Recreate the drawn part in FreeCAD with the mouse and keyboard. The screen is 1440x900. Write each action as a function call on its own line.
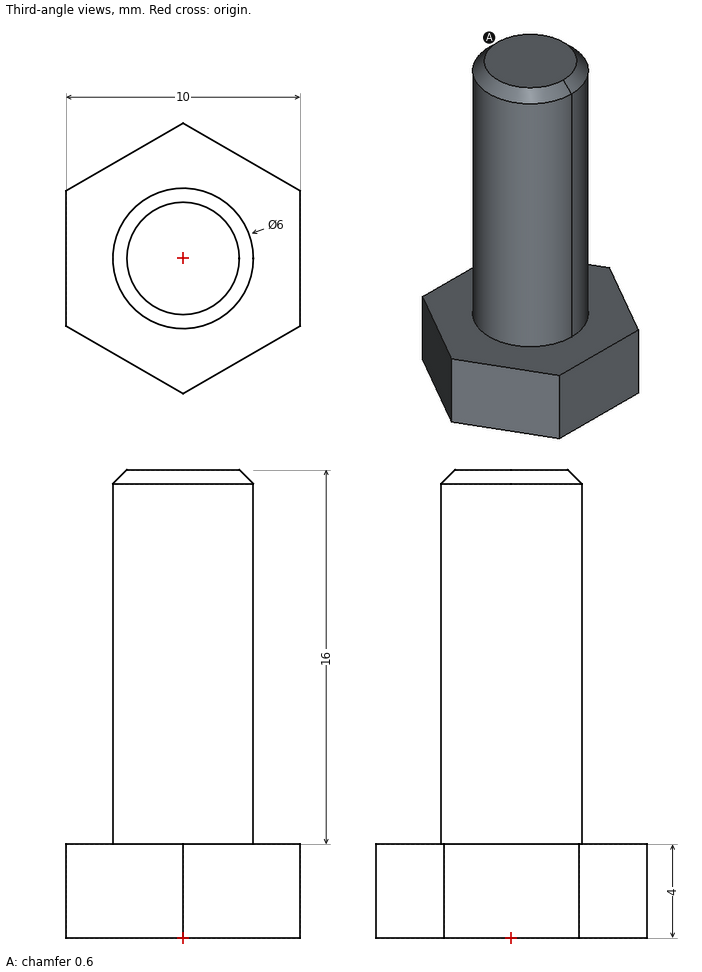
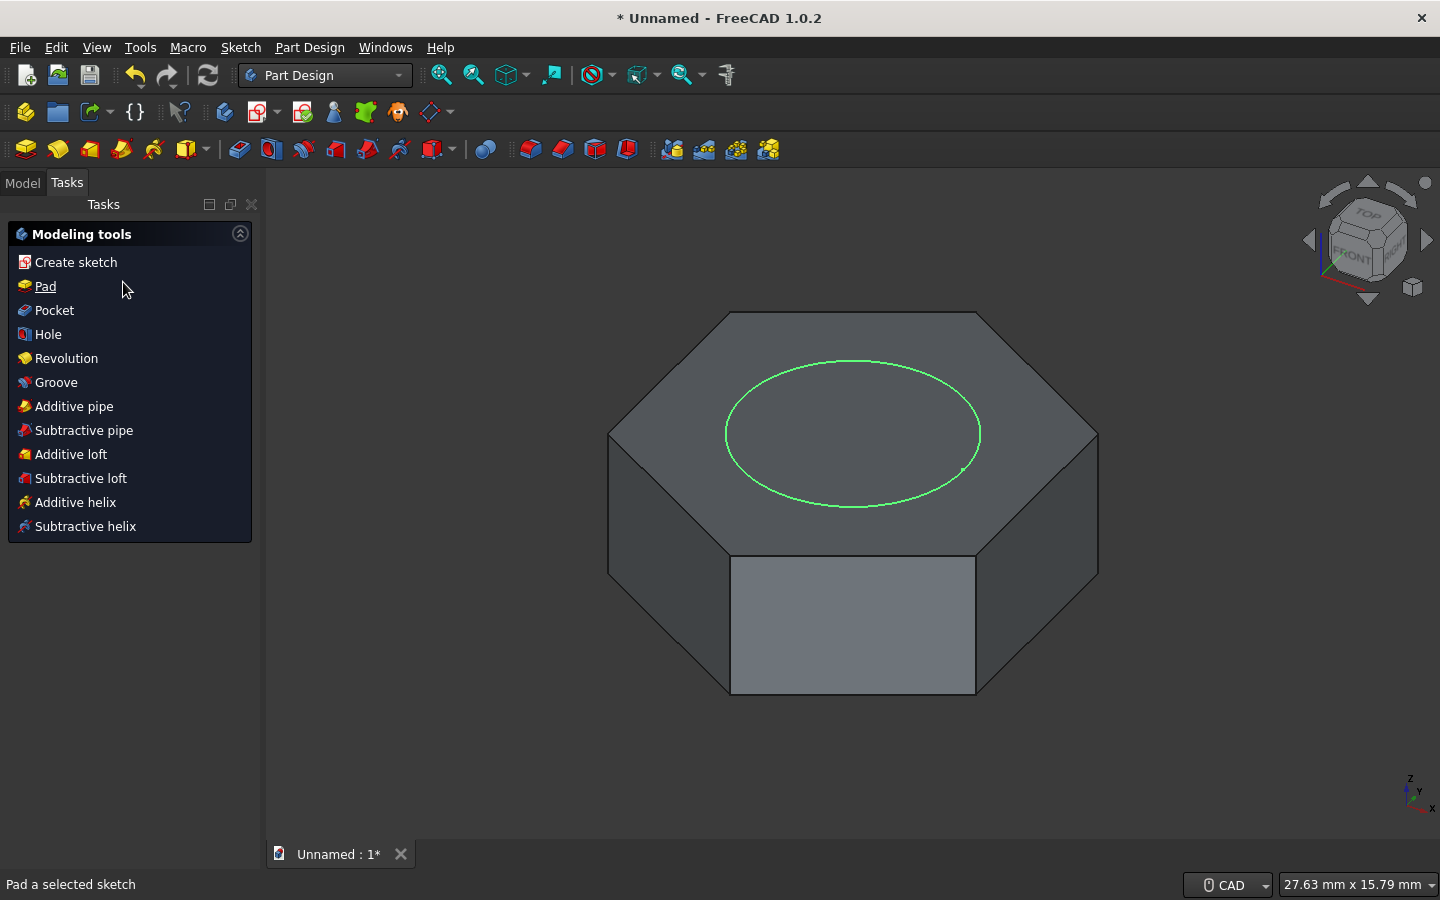
click(26, 150)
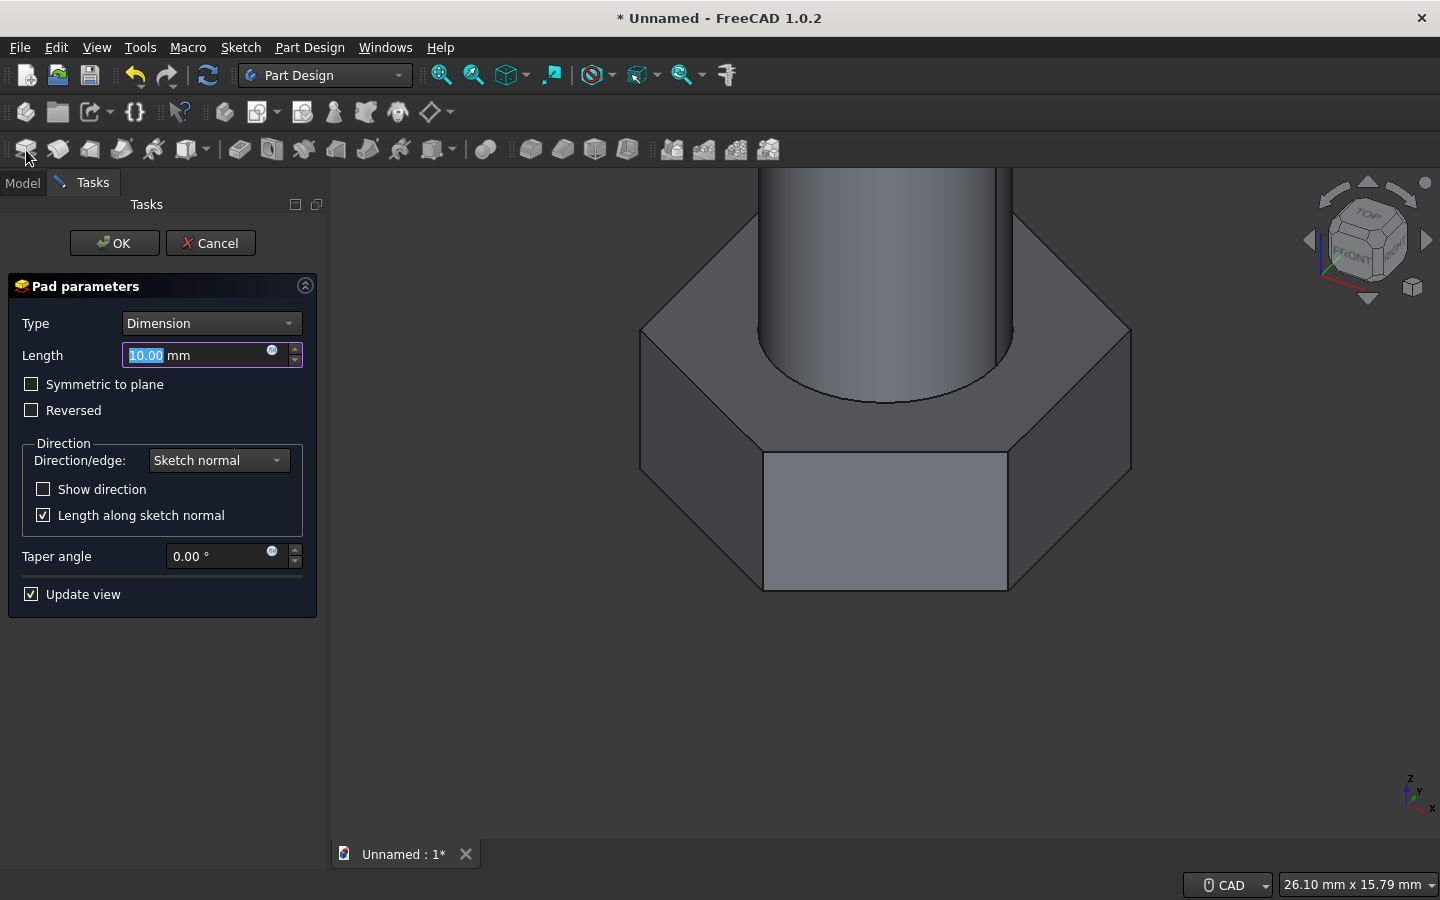
text(16)
key(Tab)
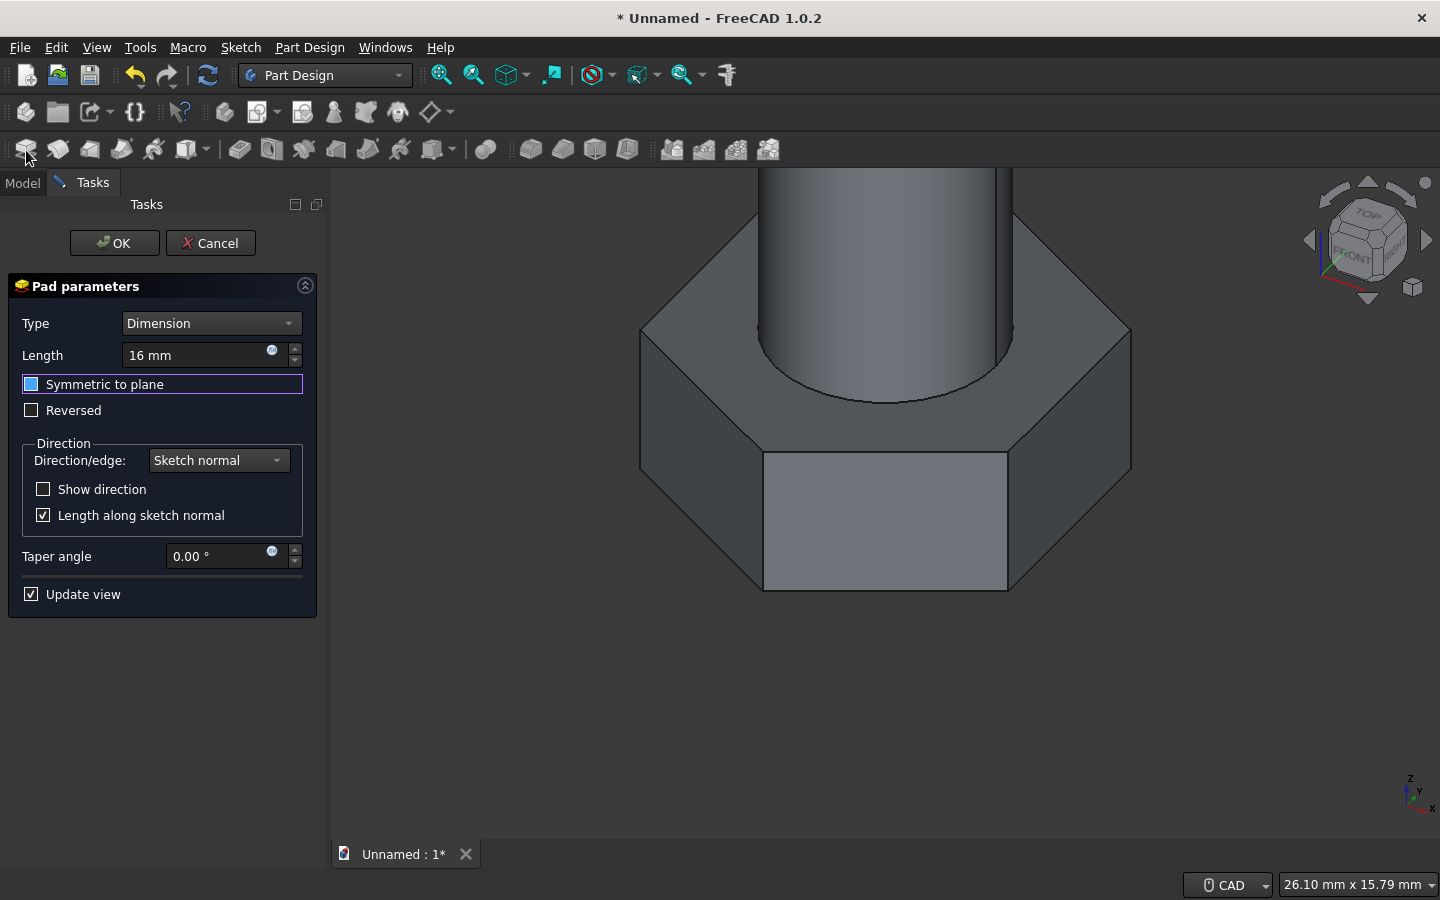
click(115, 243)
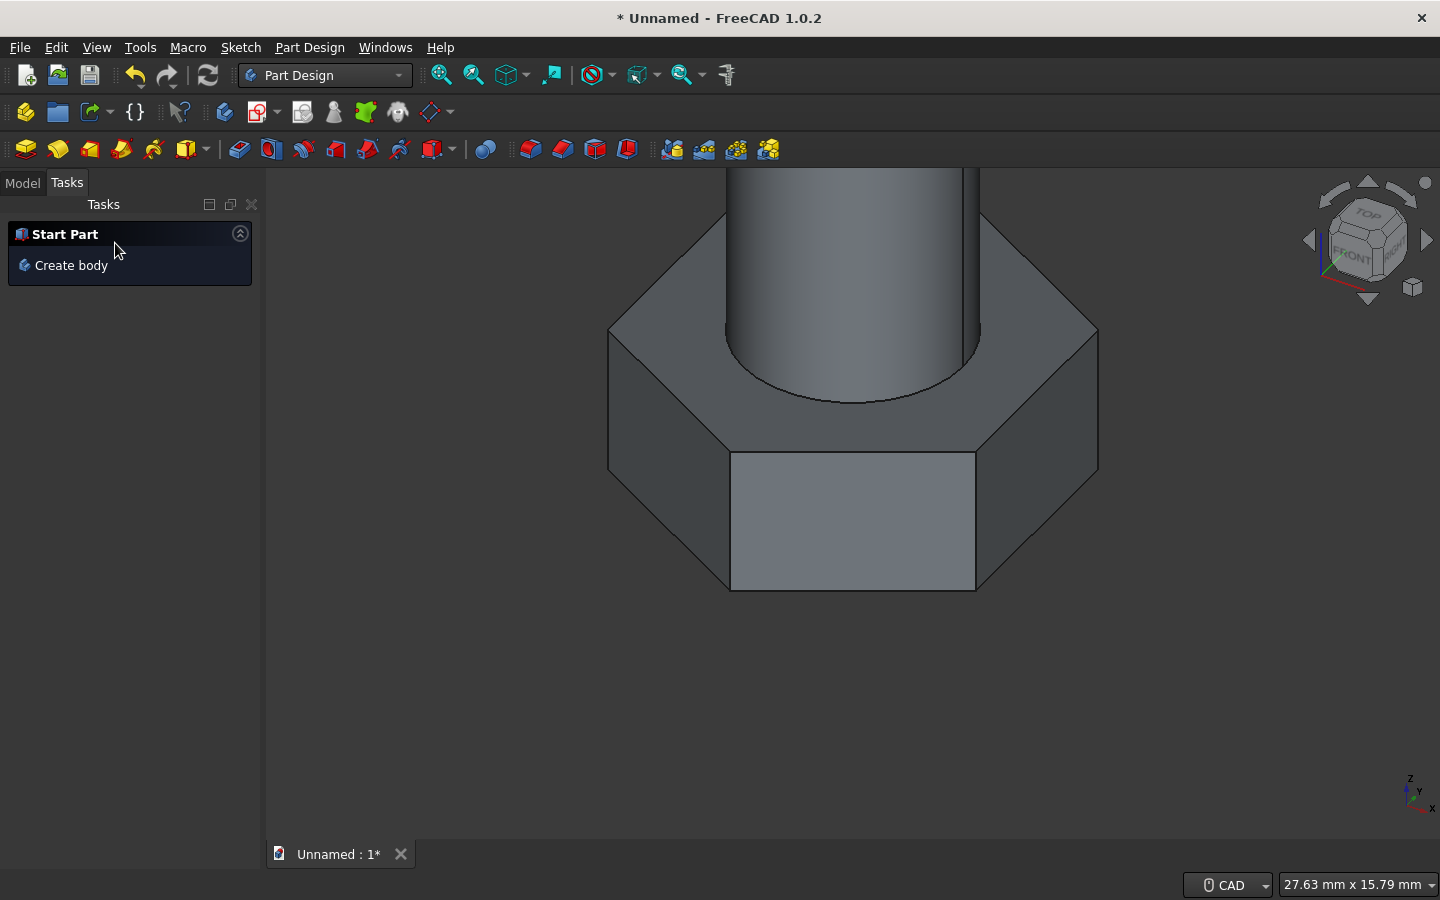
click(442, 76)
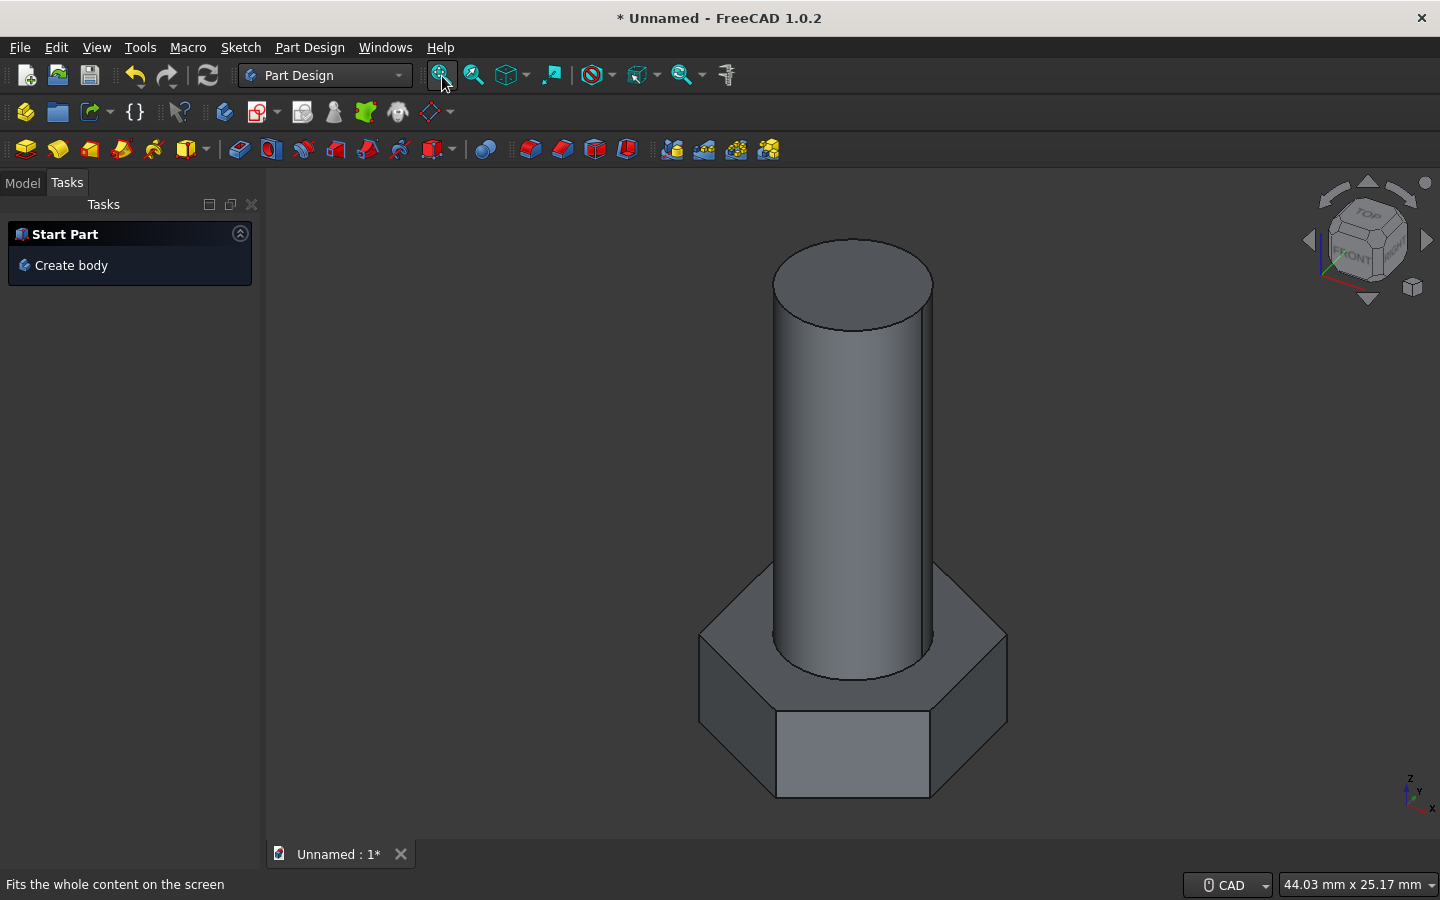
click(773, 289)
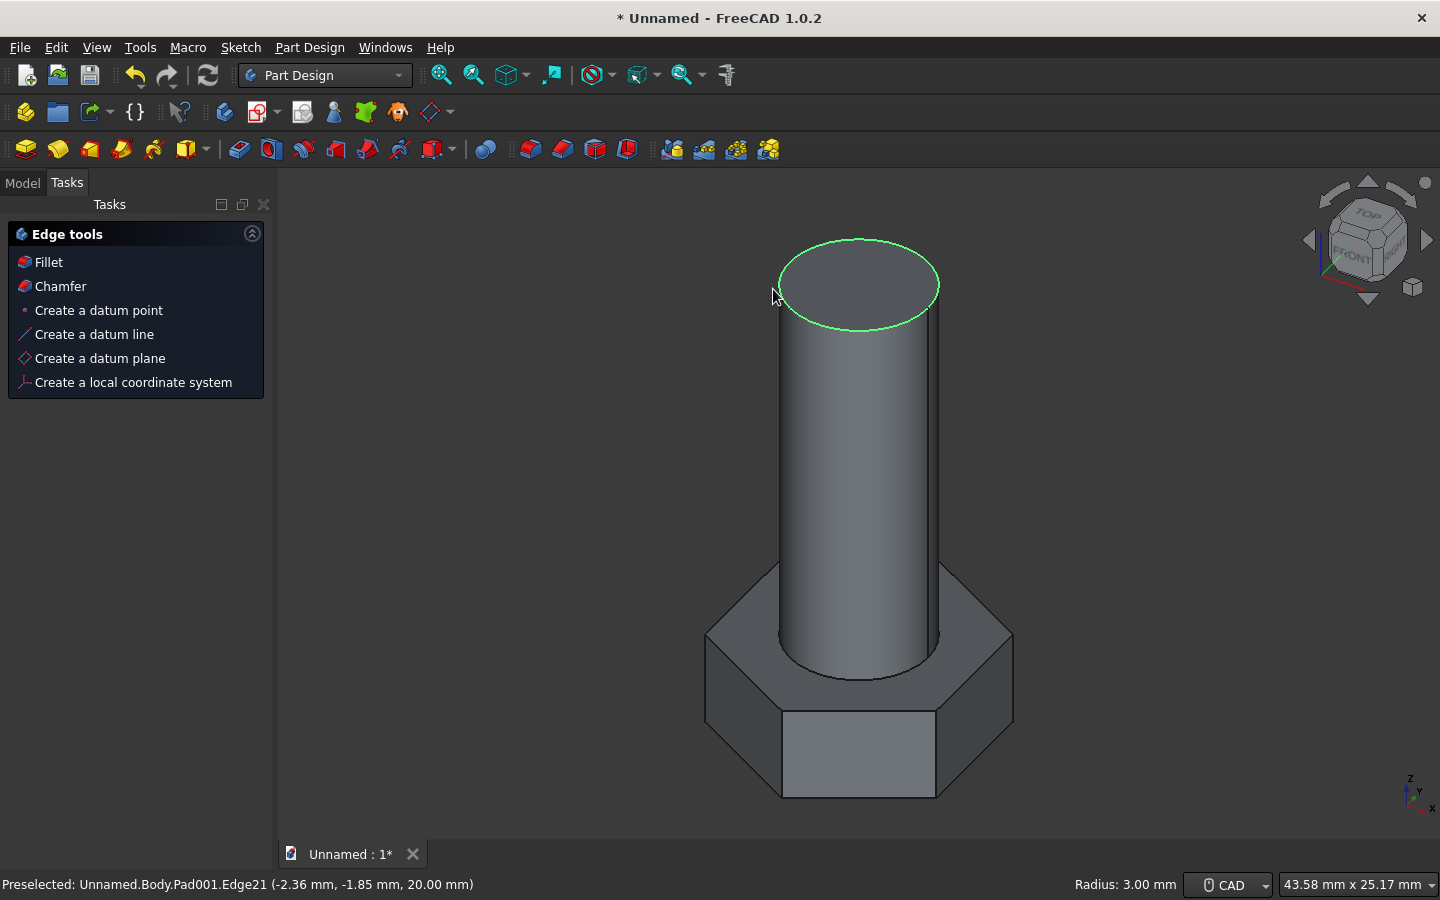
click(564, 150)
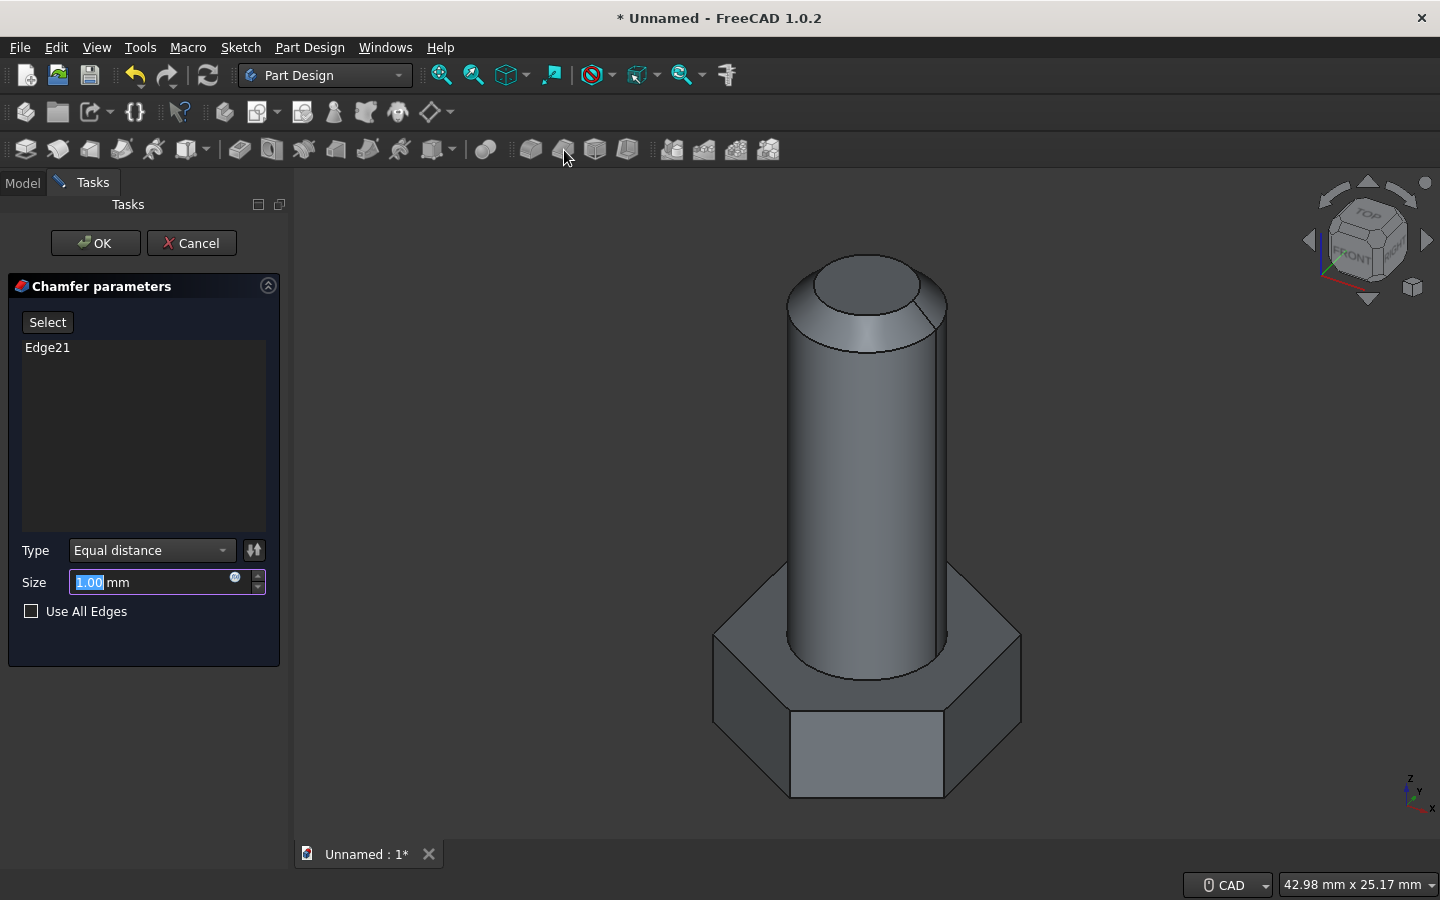
text(0.6)
key(Tab)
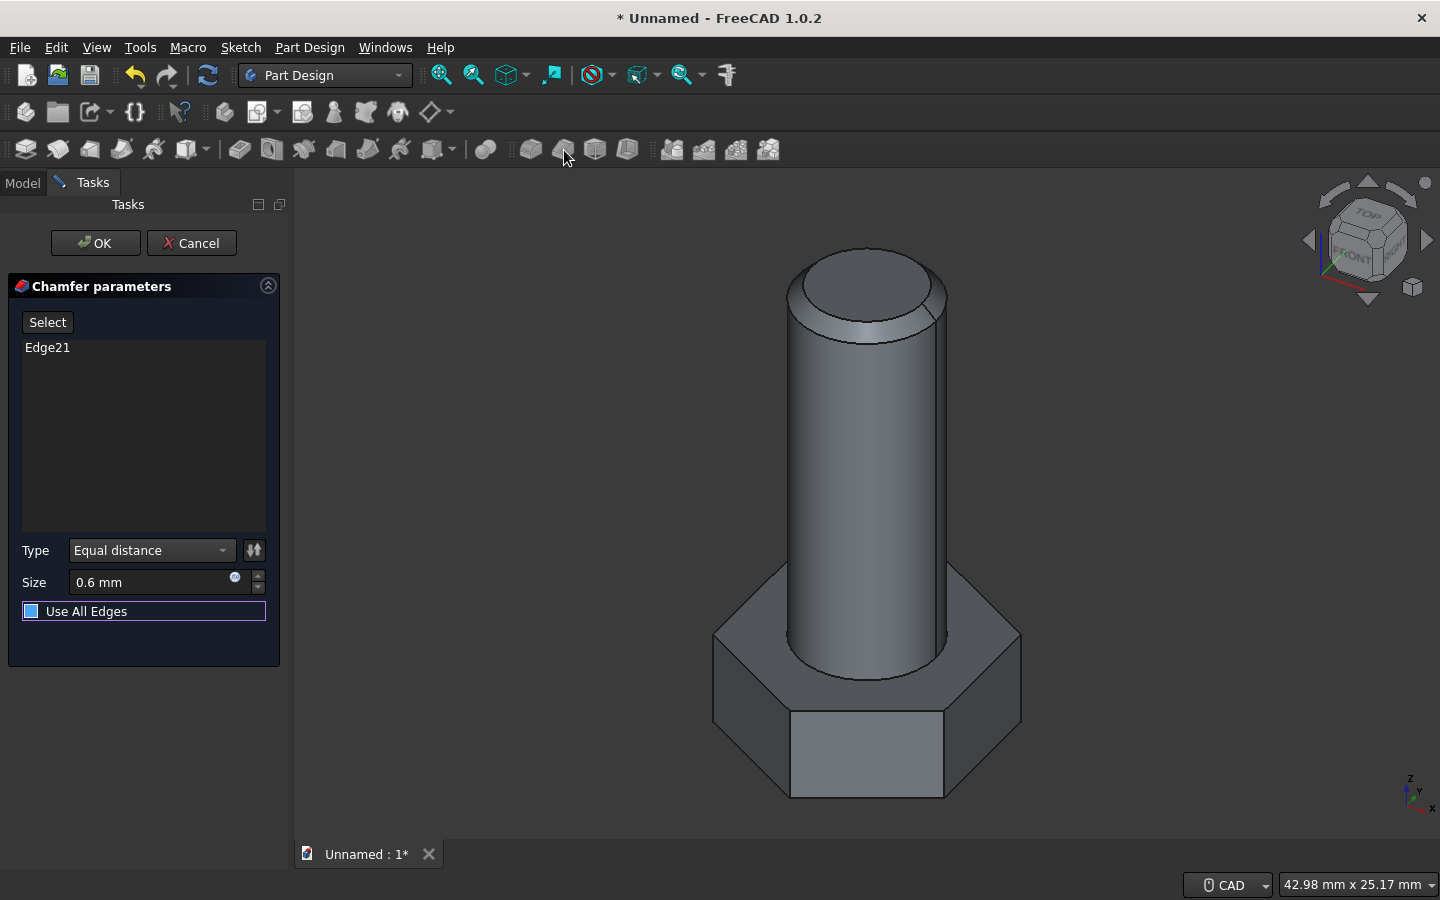
click(96, 243)